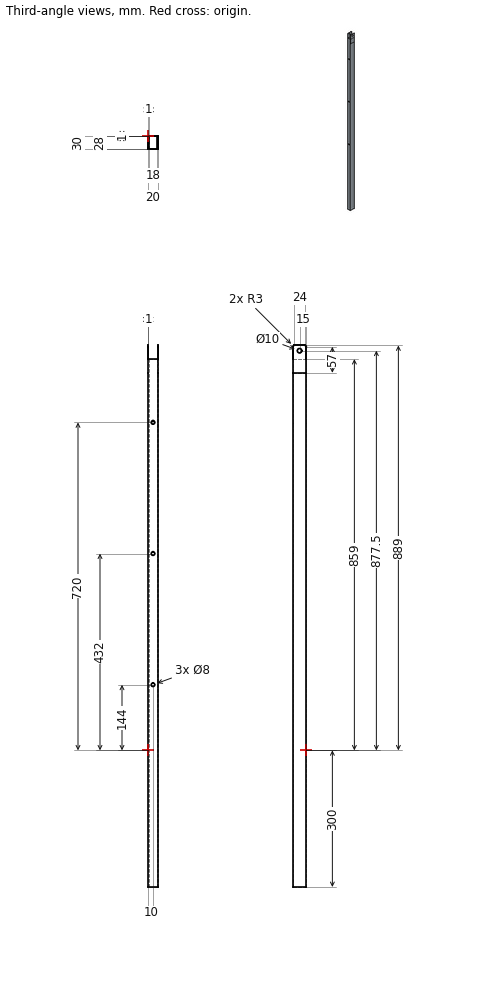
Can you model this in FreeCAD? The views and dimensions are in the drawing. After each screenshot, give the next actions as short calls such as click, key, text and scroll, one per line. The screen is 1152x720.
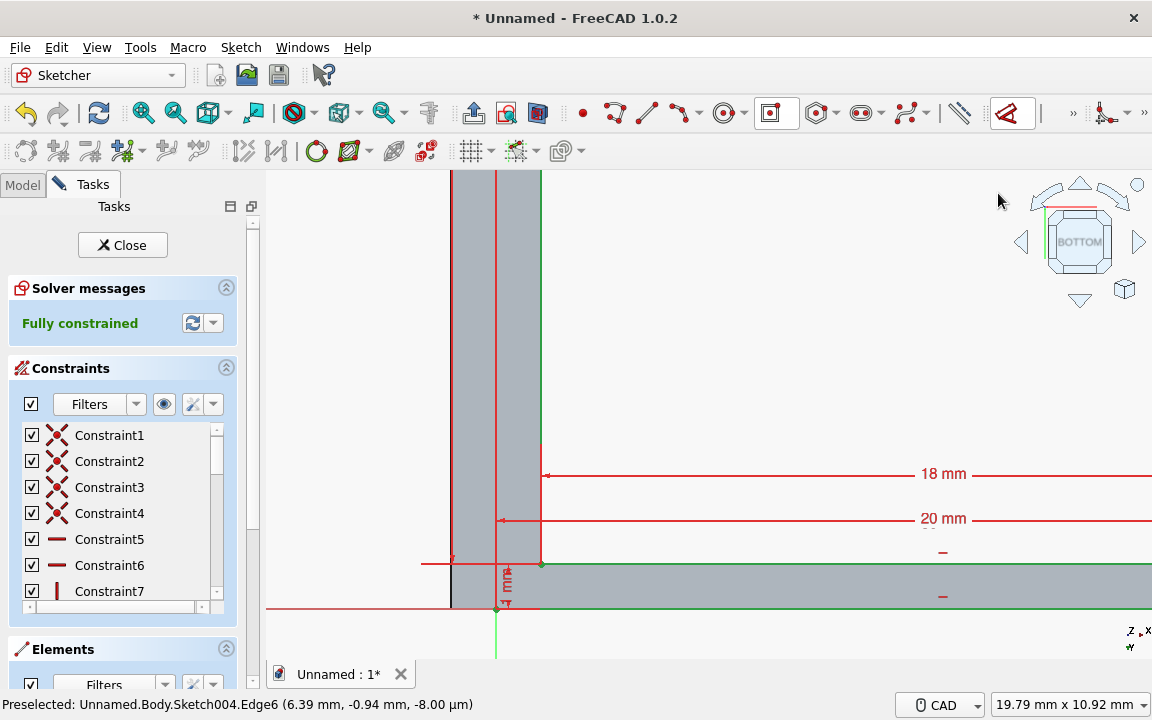
click(123, 245)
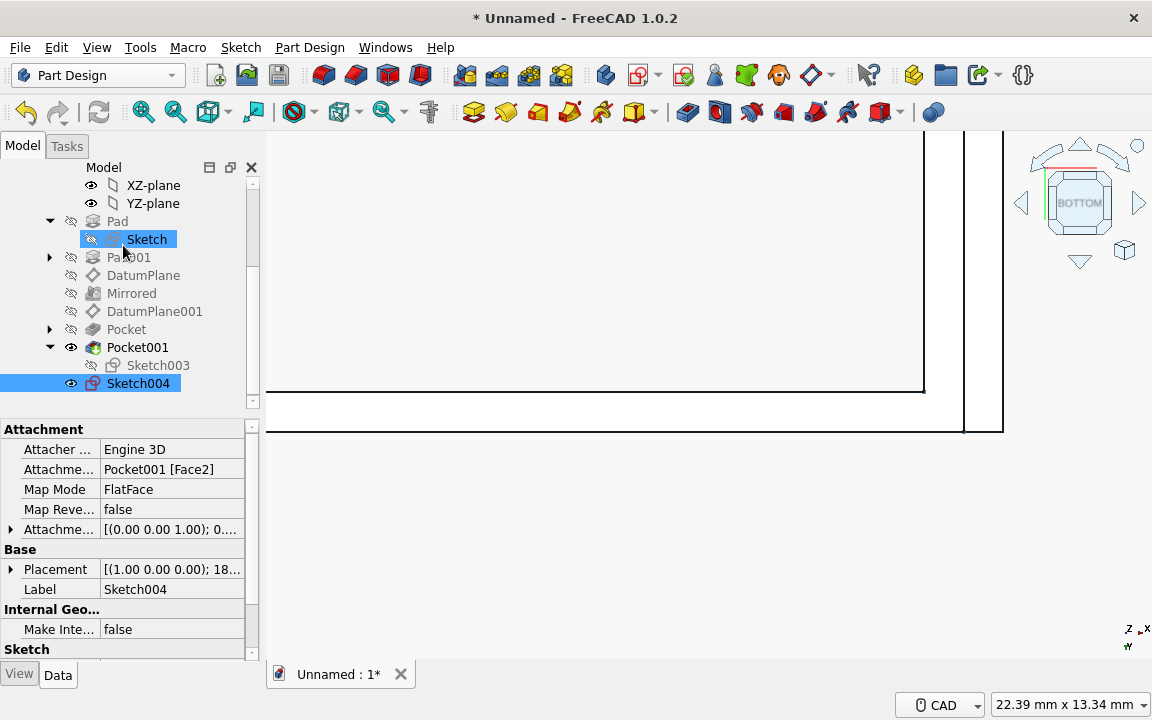
click(474, 112)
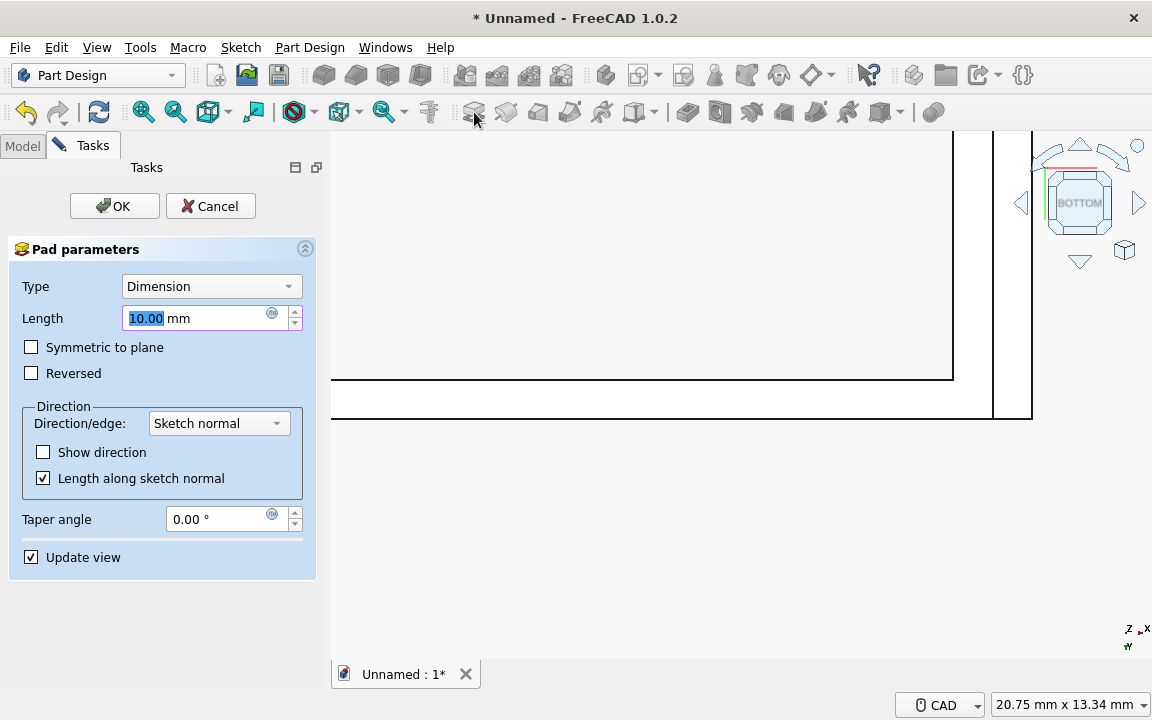
text(300)
key(Tab)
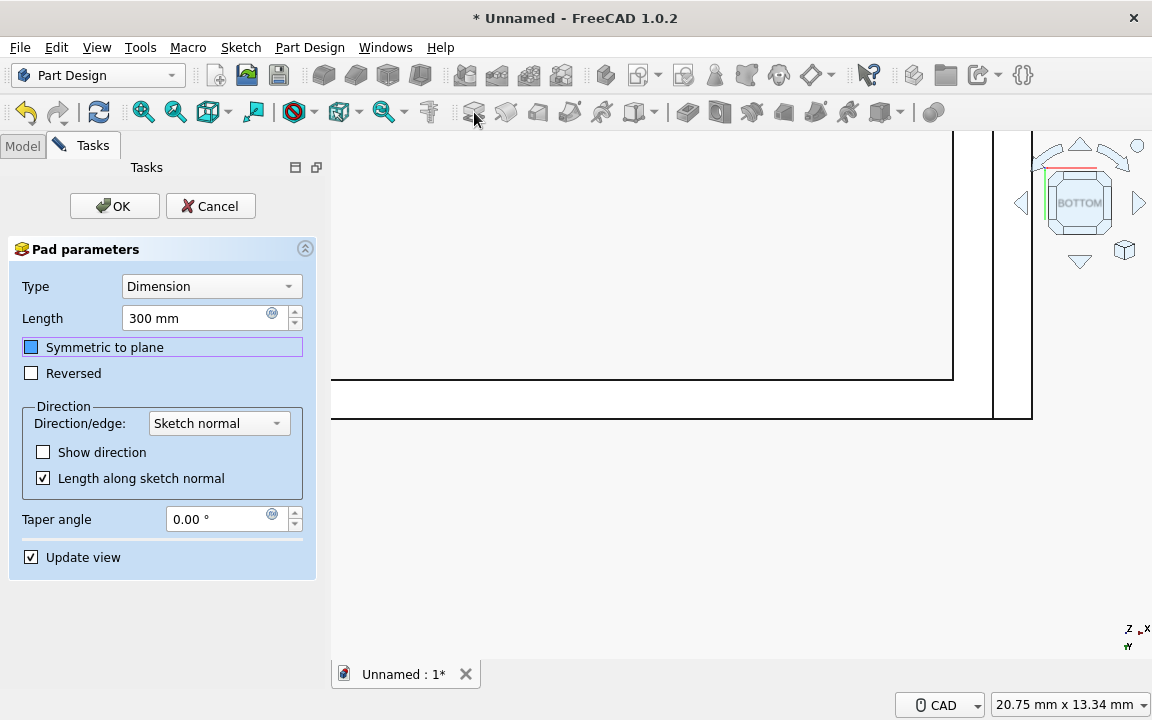
click(115, 206)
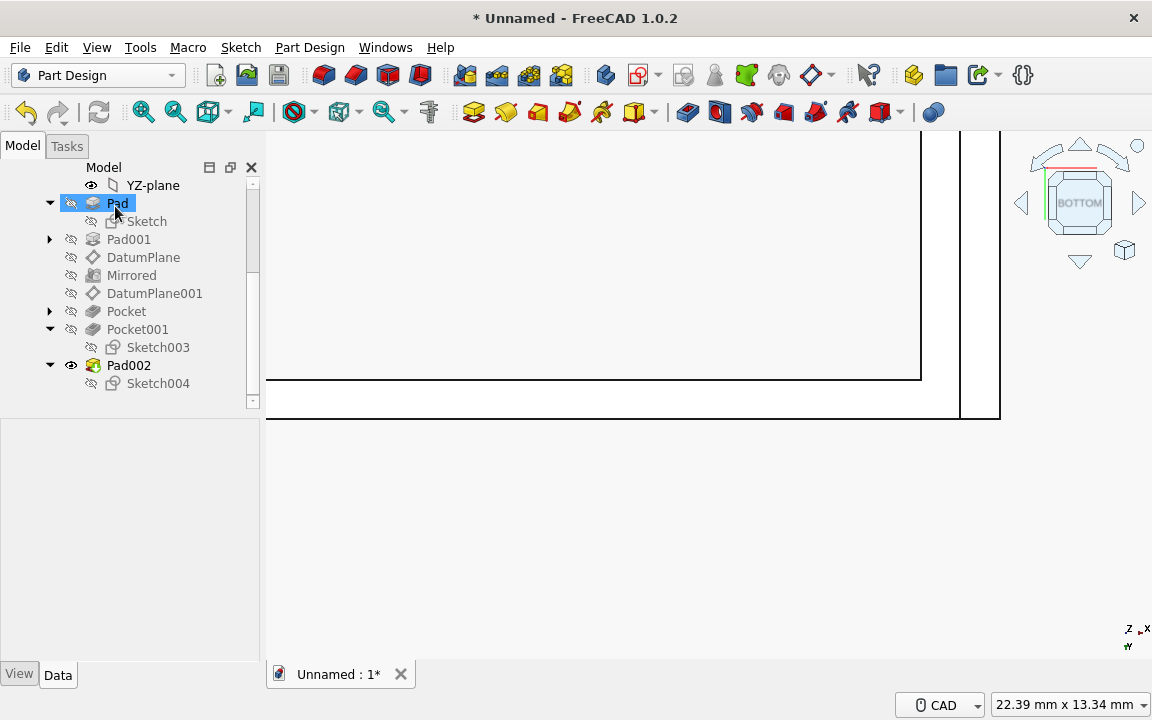
key(0)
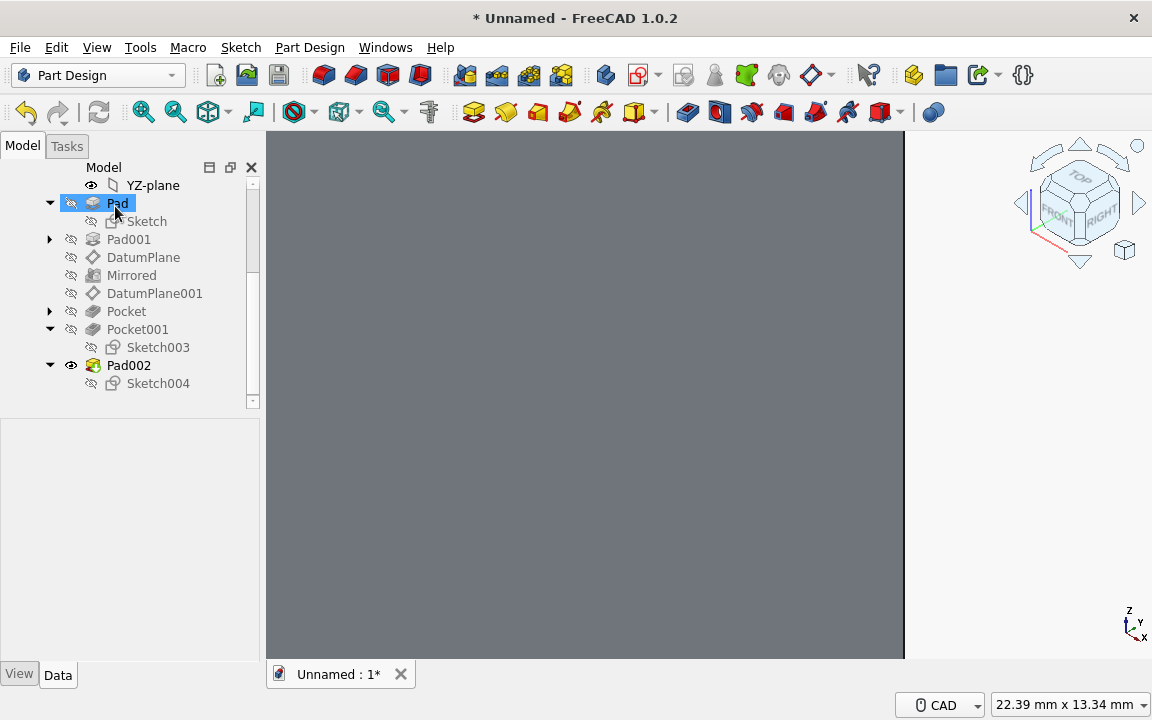
key(v)
key(f)